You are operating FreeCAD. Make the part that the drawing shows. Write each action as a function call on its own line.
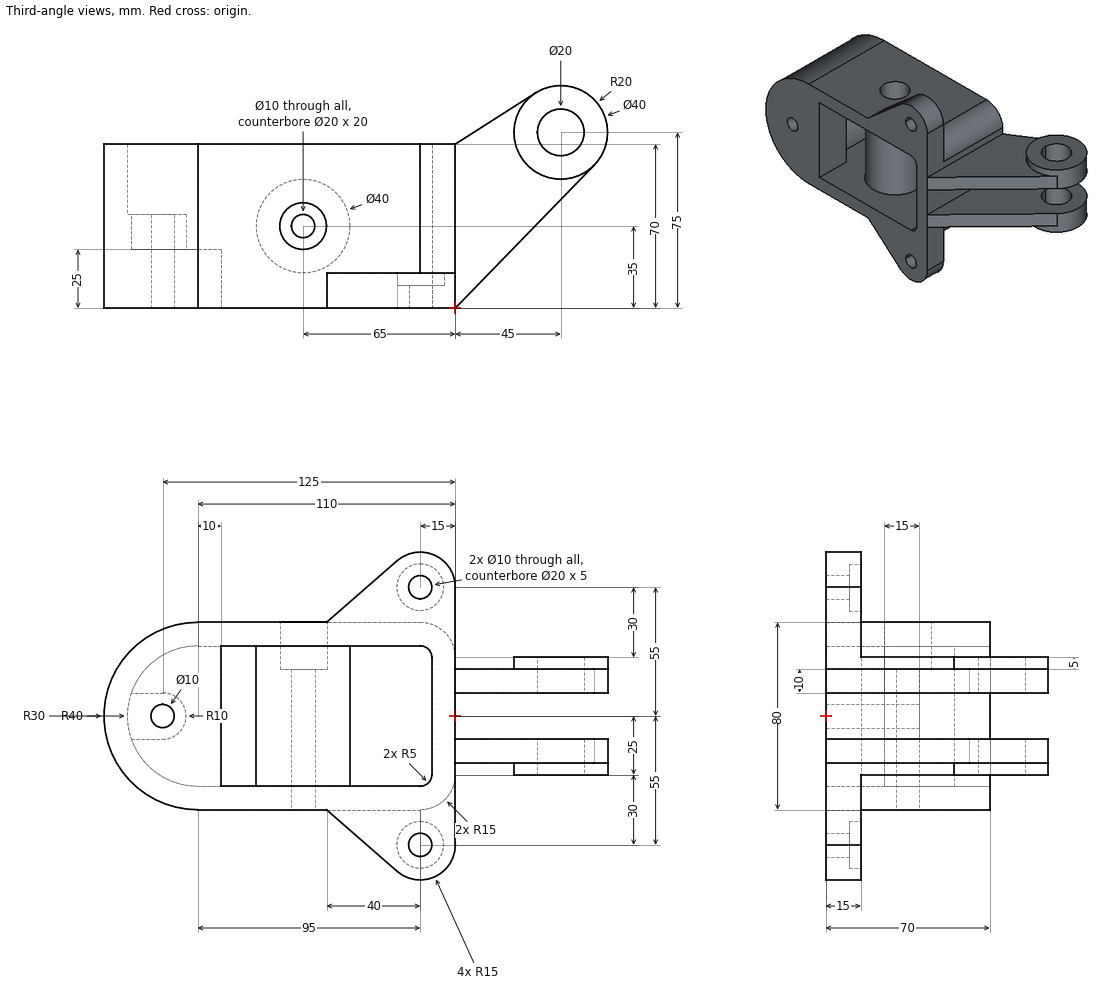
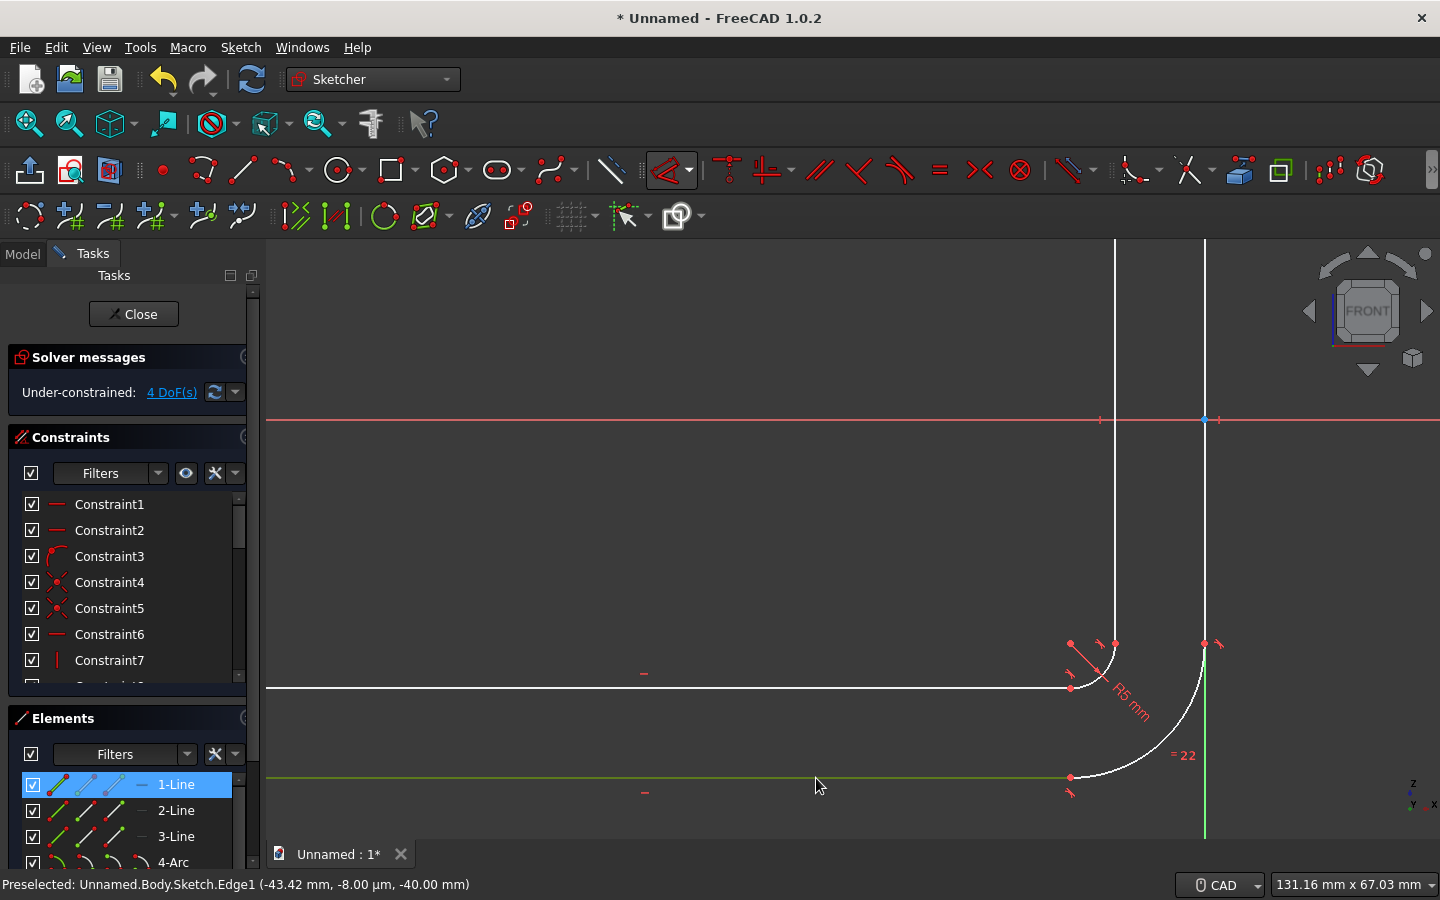
key(l)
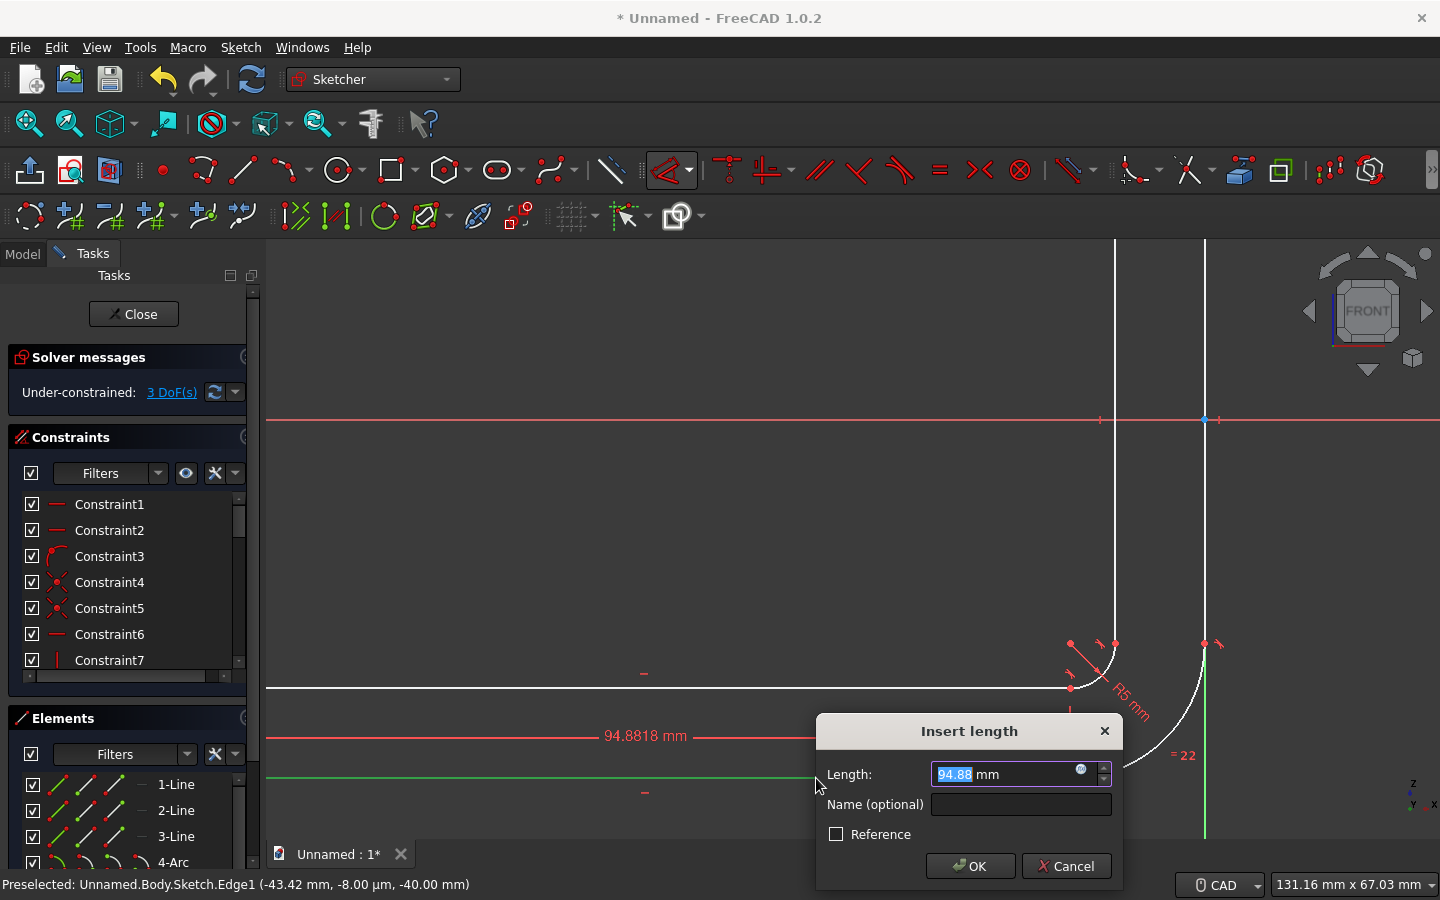
text(95)
key(Return)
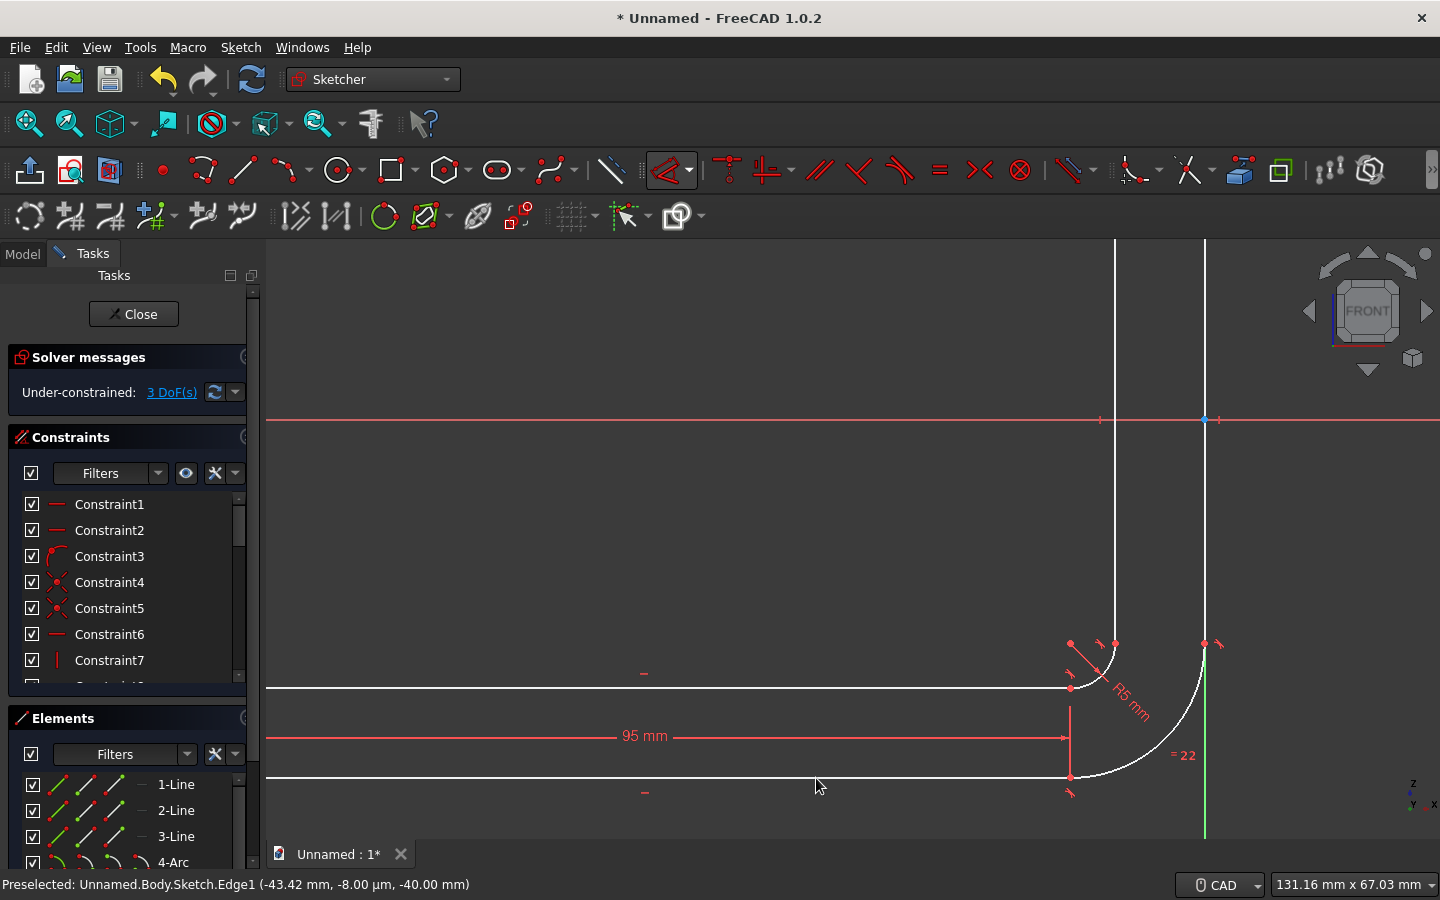
scroll(1090, 684, down, 3)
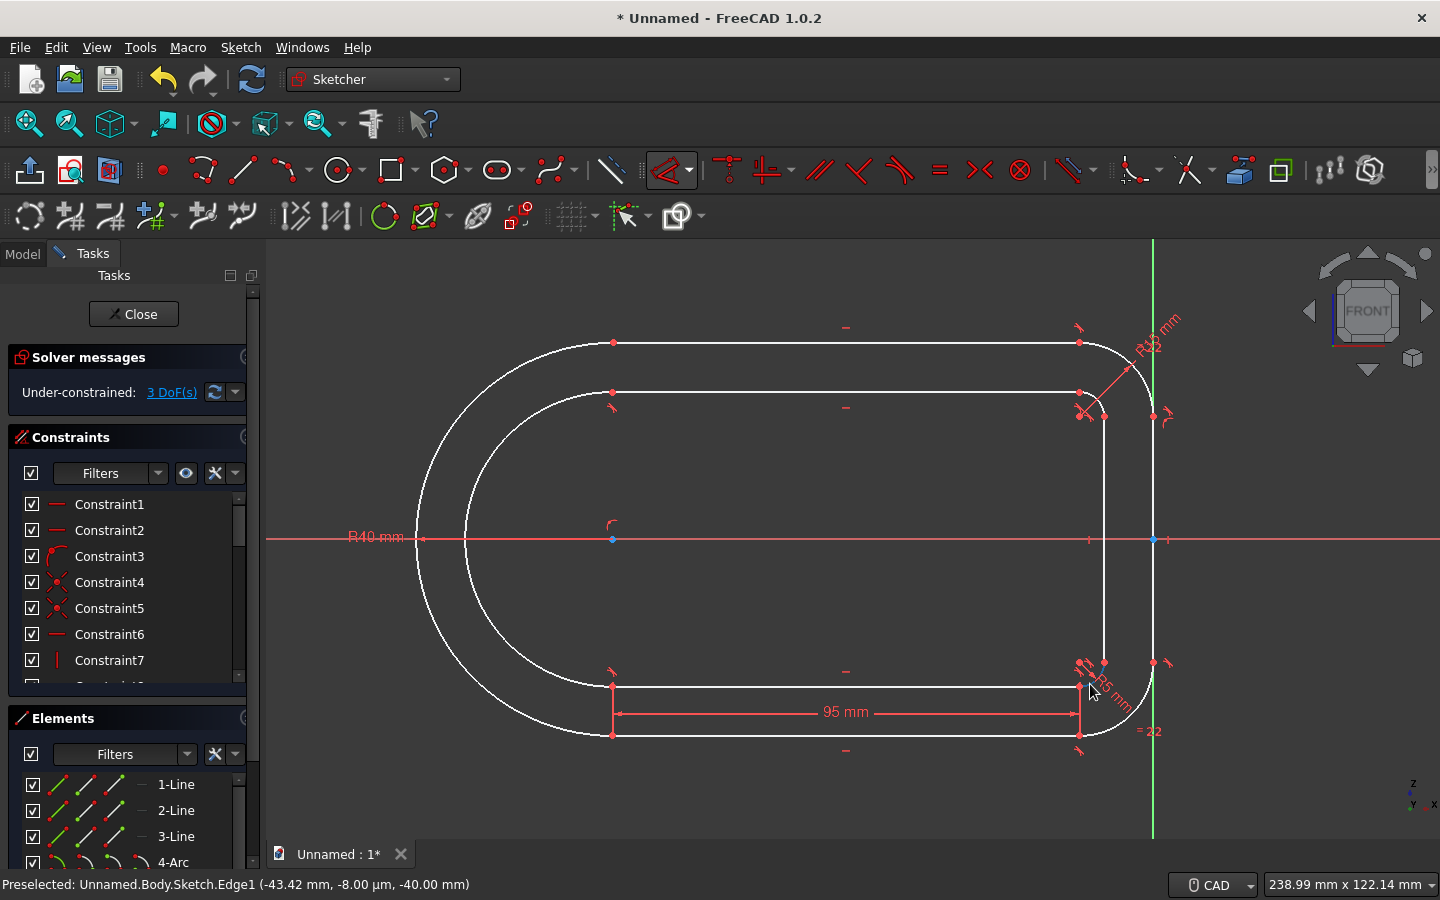
click(753, 343)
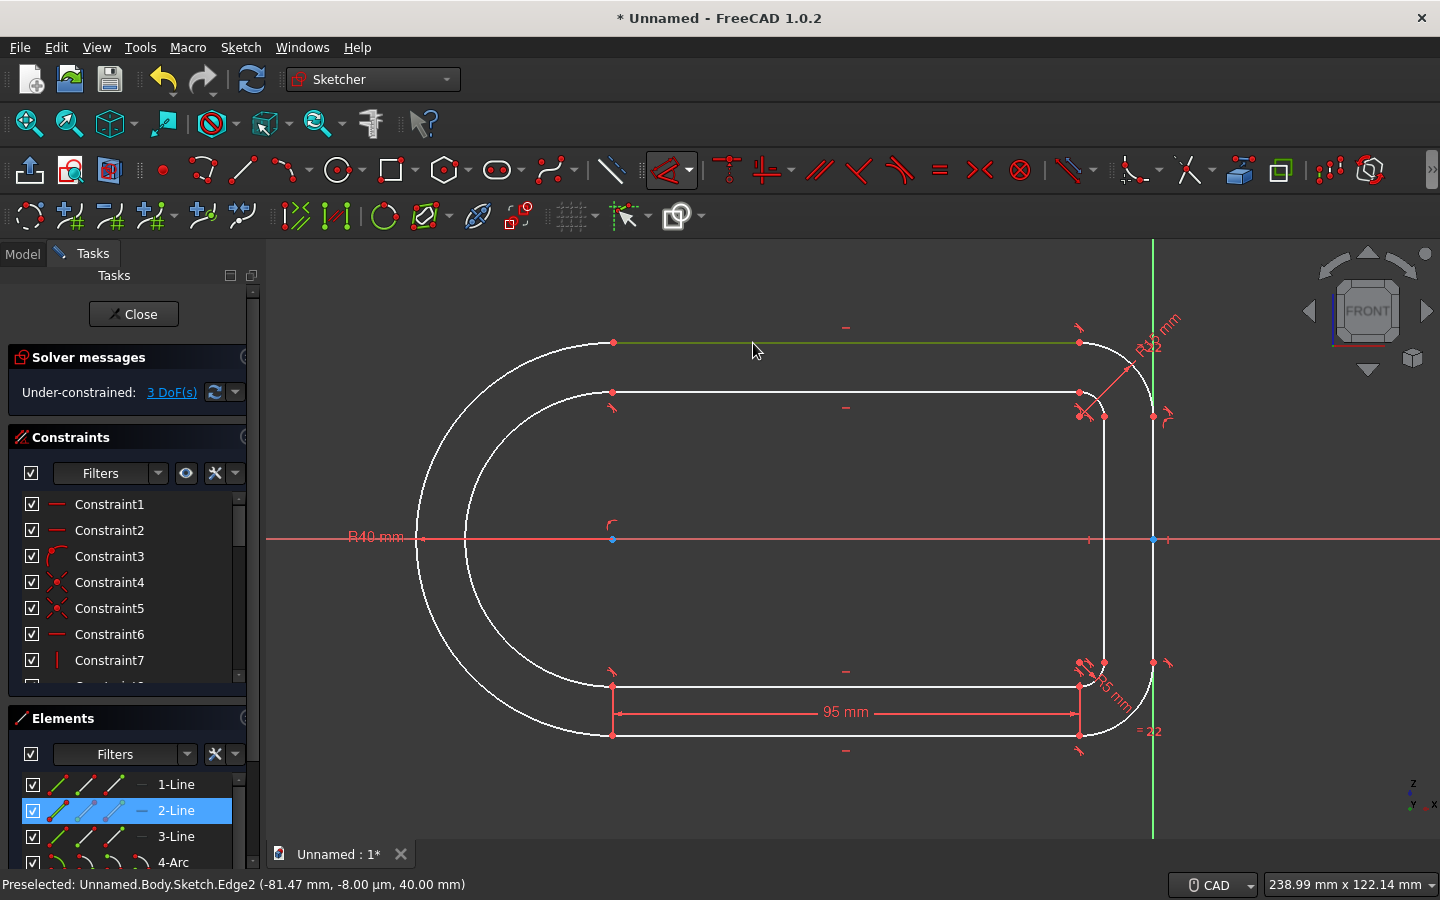
key(l)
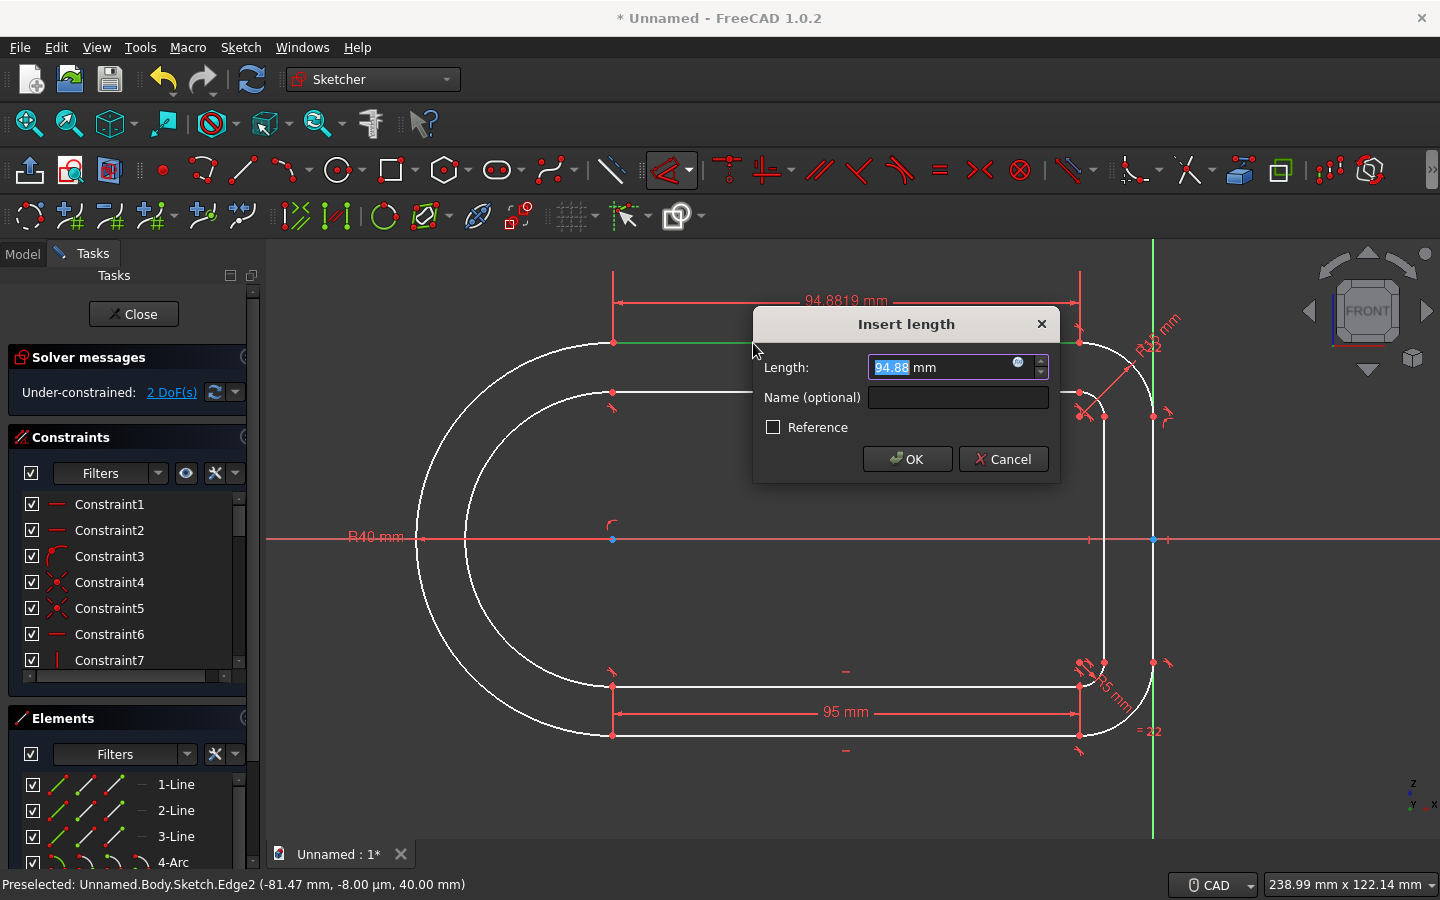
text(95)
key(Return)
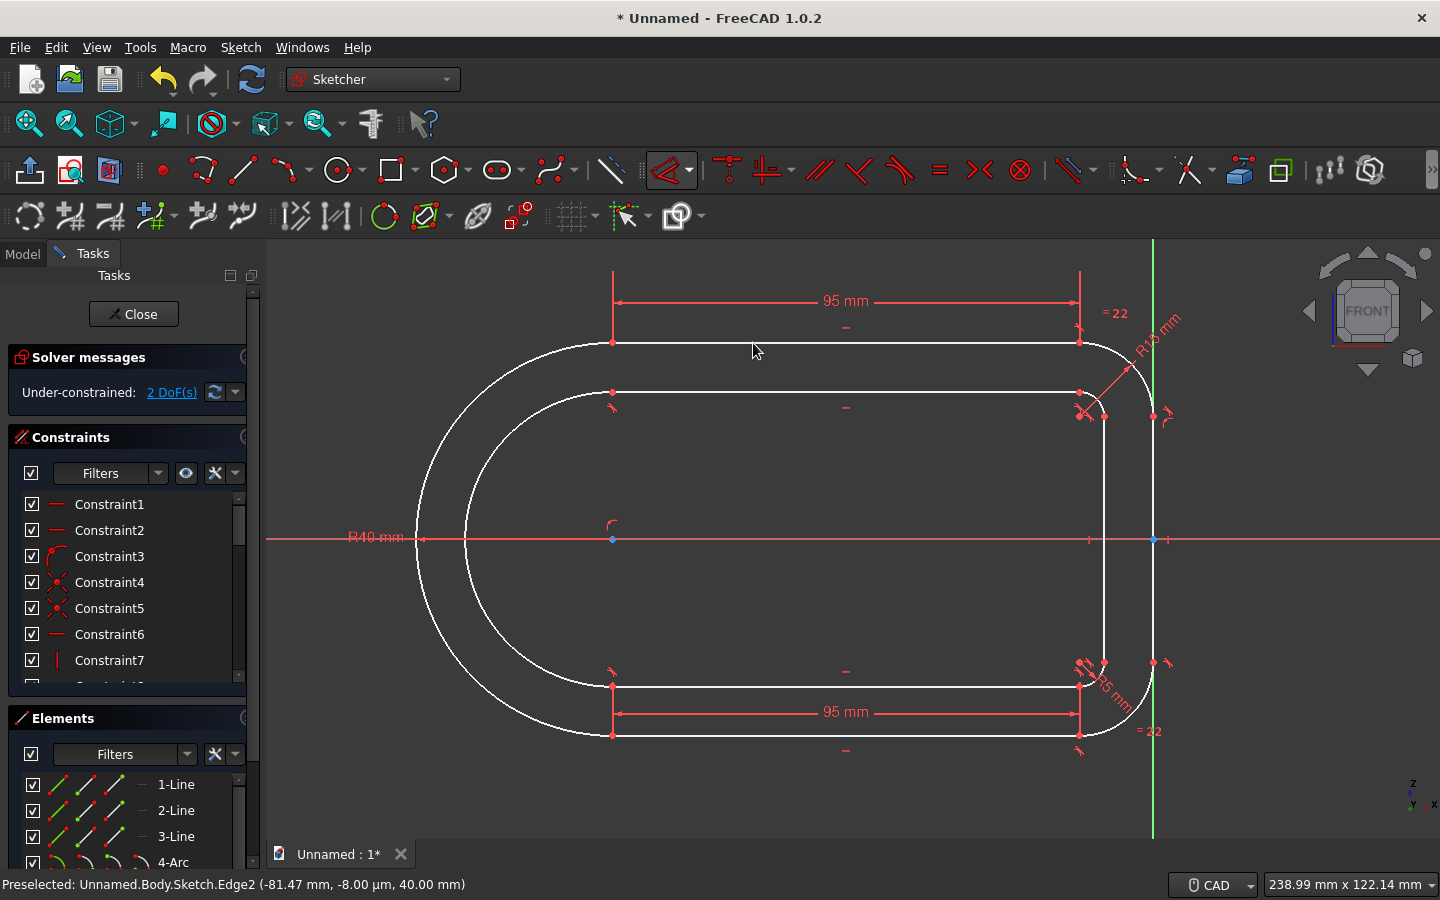
click(753, 687)